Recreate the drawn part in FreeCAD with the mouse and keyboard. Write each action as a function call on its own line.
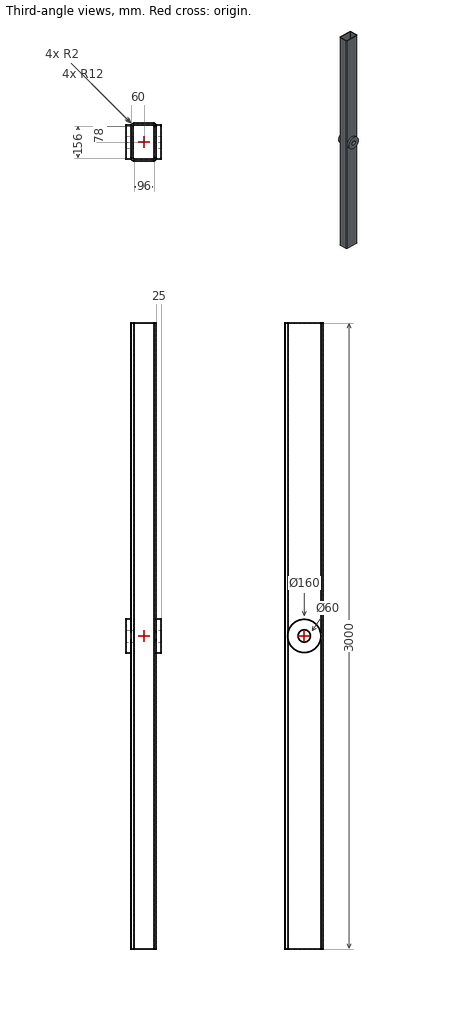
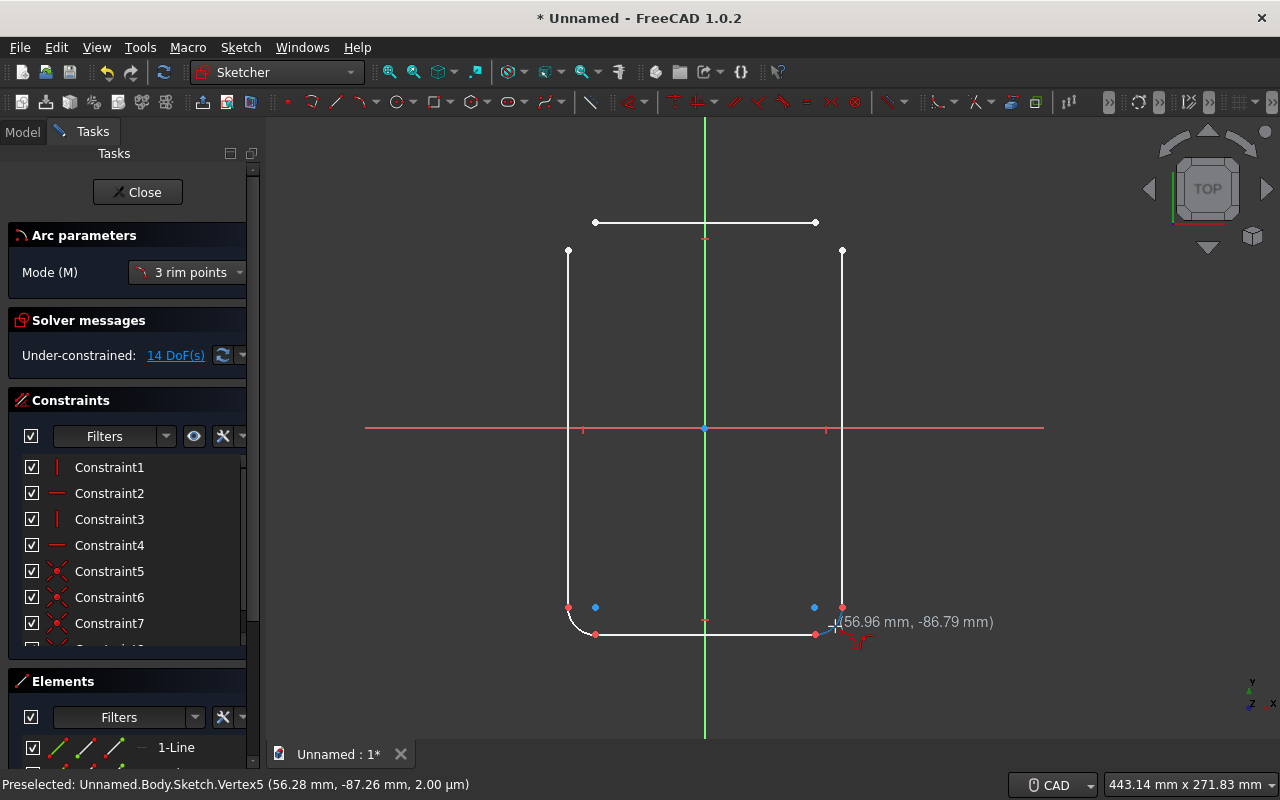
click(842, 251)
click(815, 223)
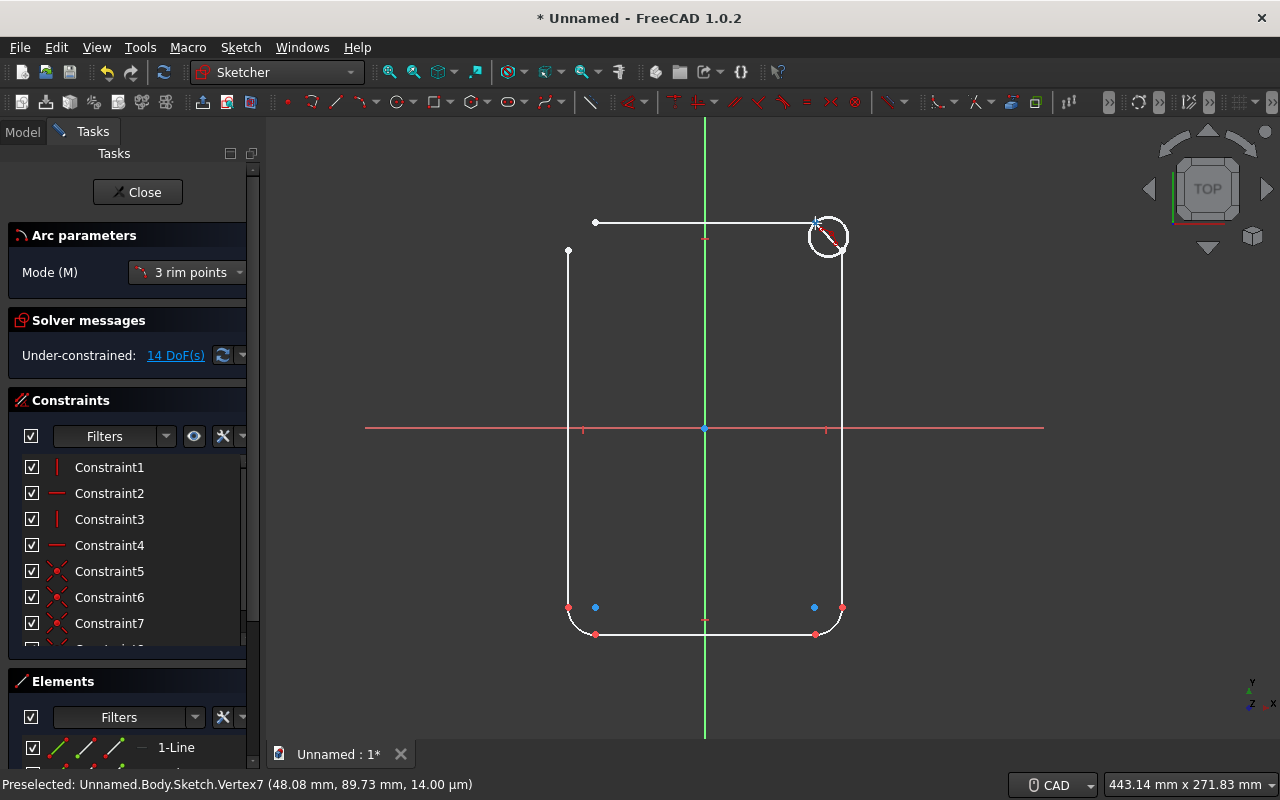
scroll(834, 230, up, 4)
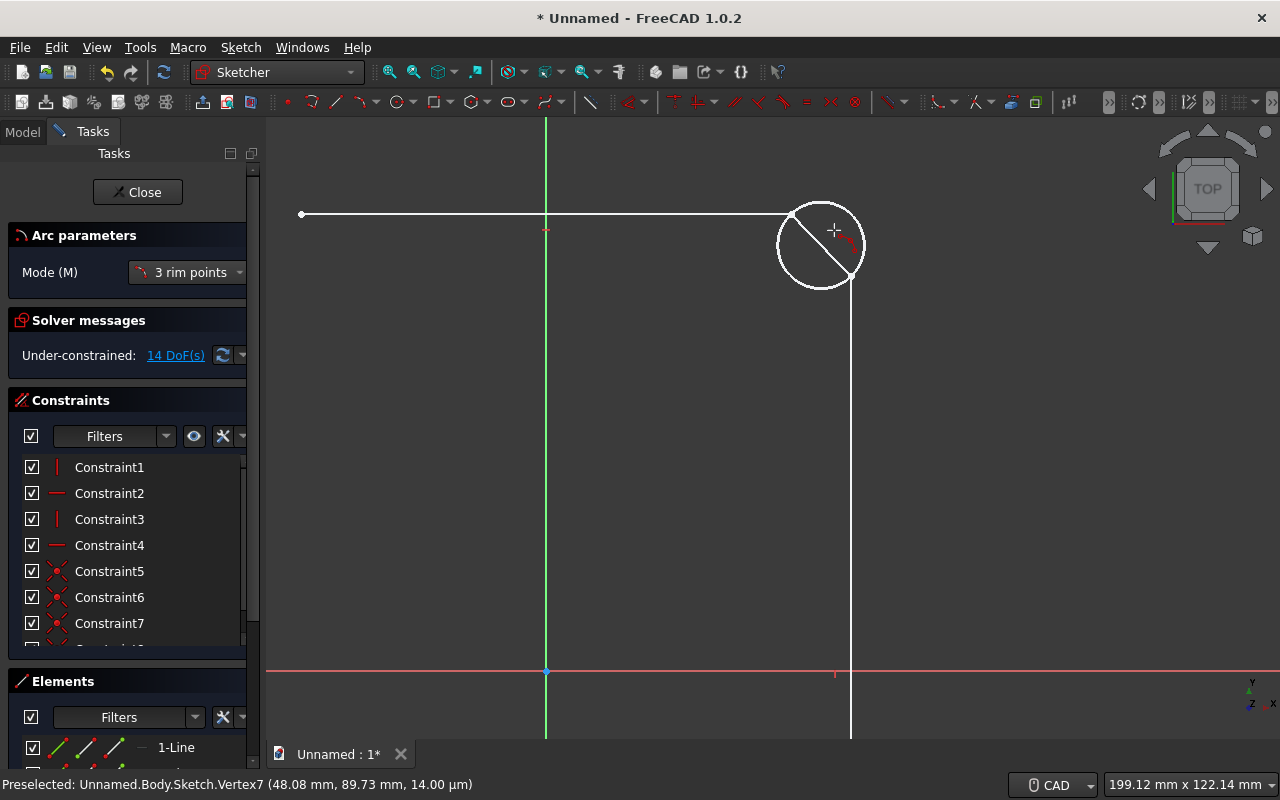
click(834, 231)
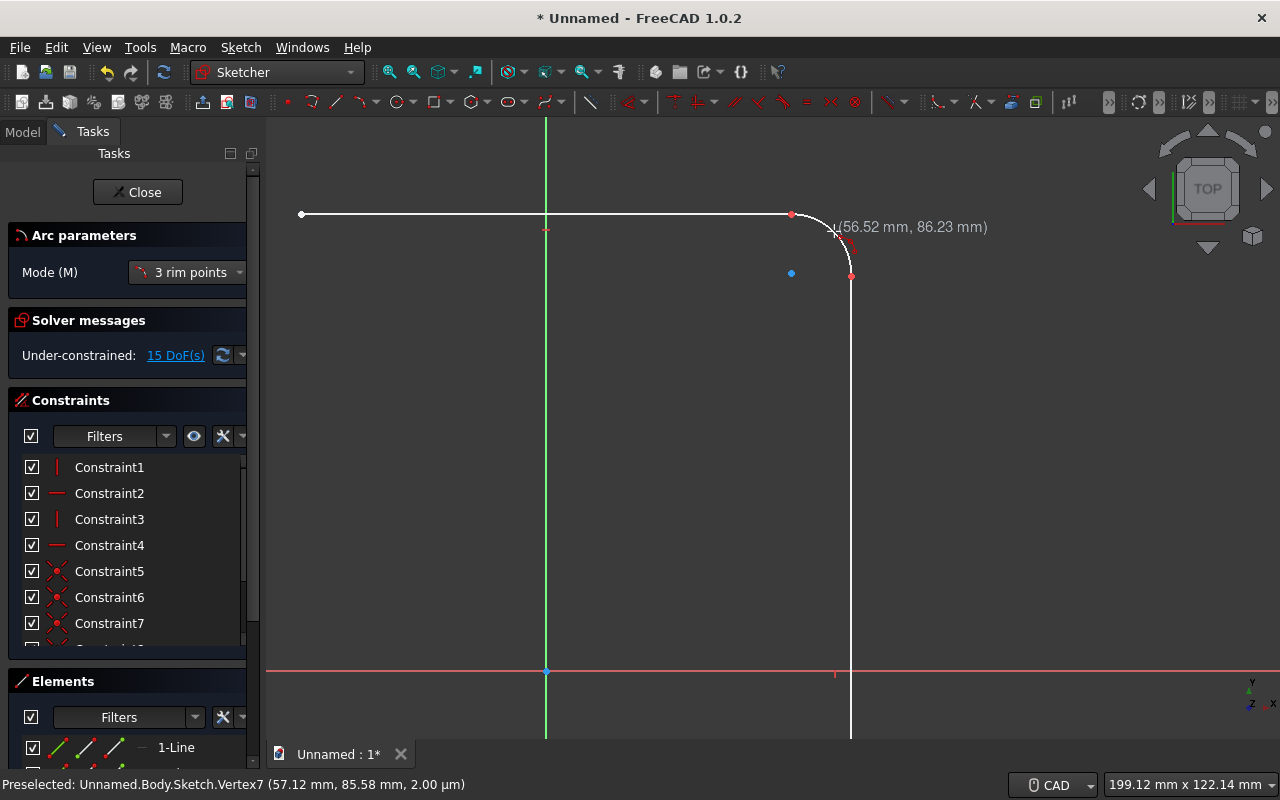
click(301, 214)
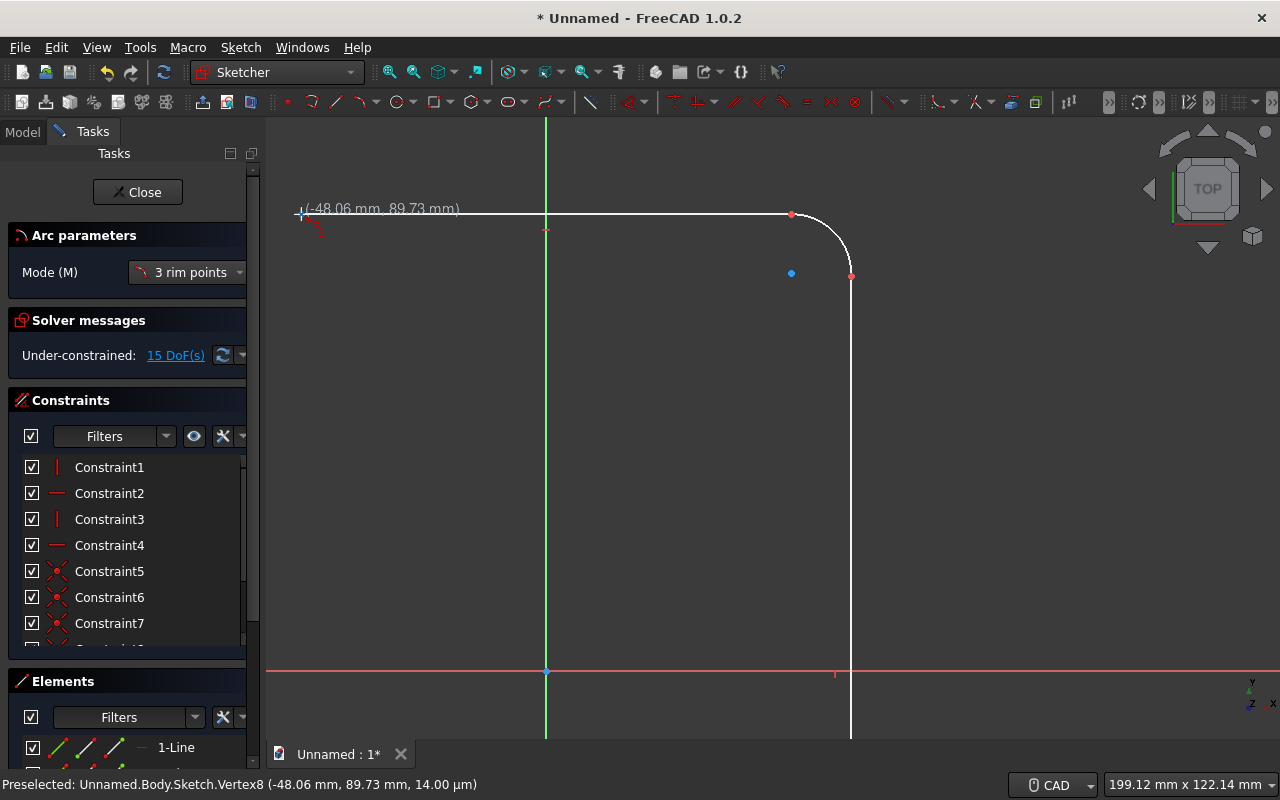
scroll(834, 230, down, 4)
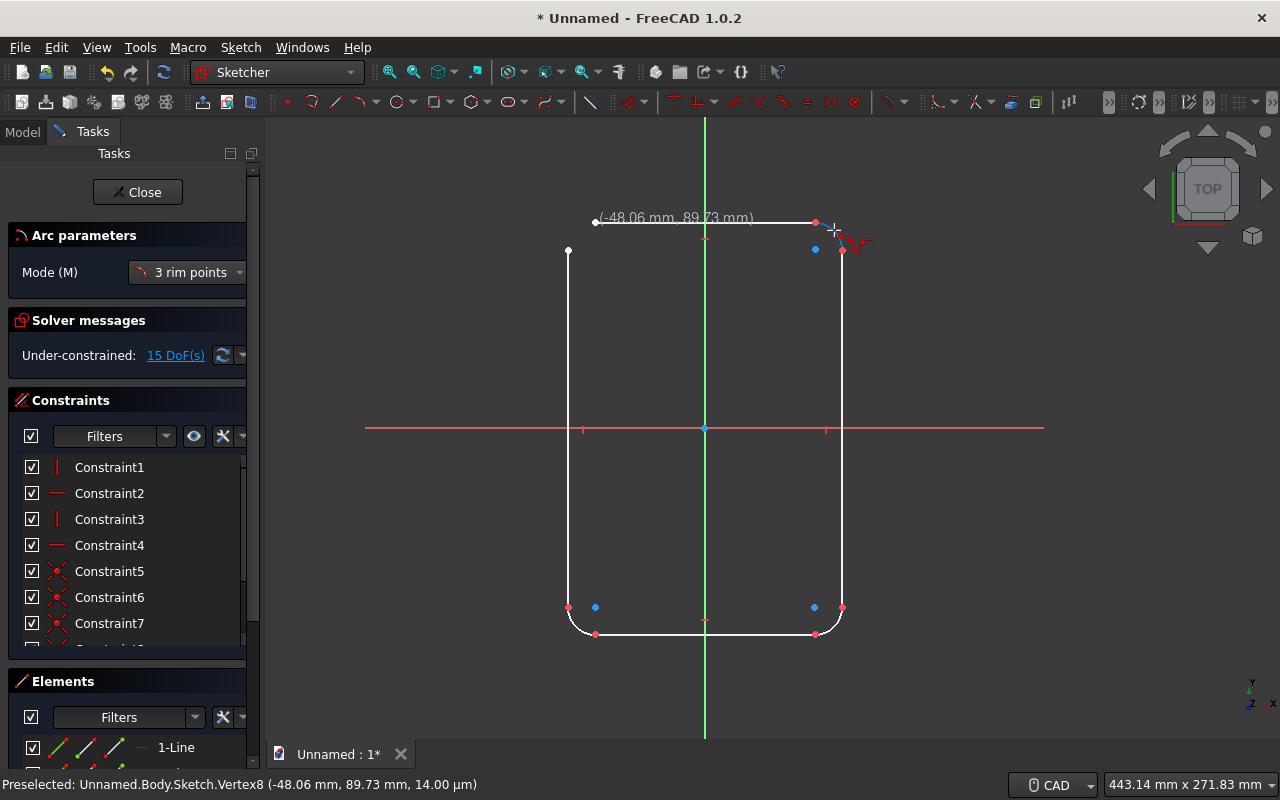
click(568, 251)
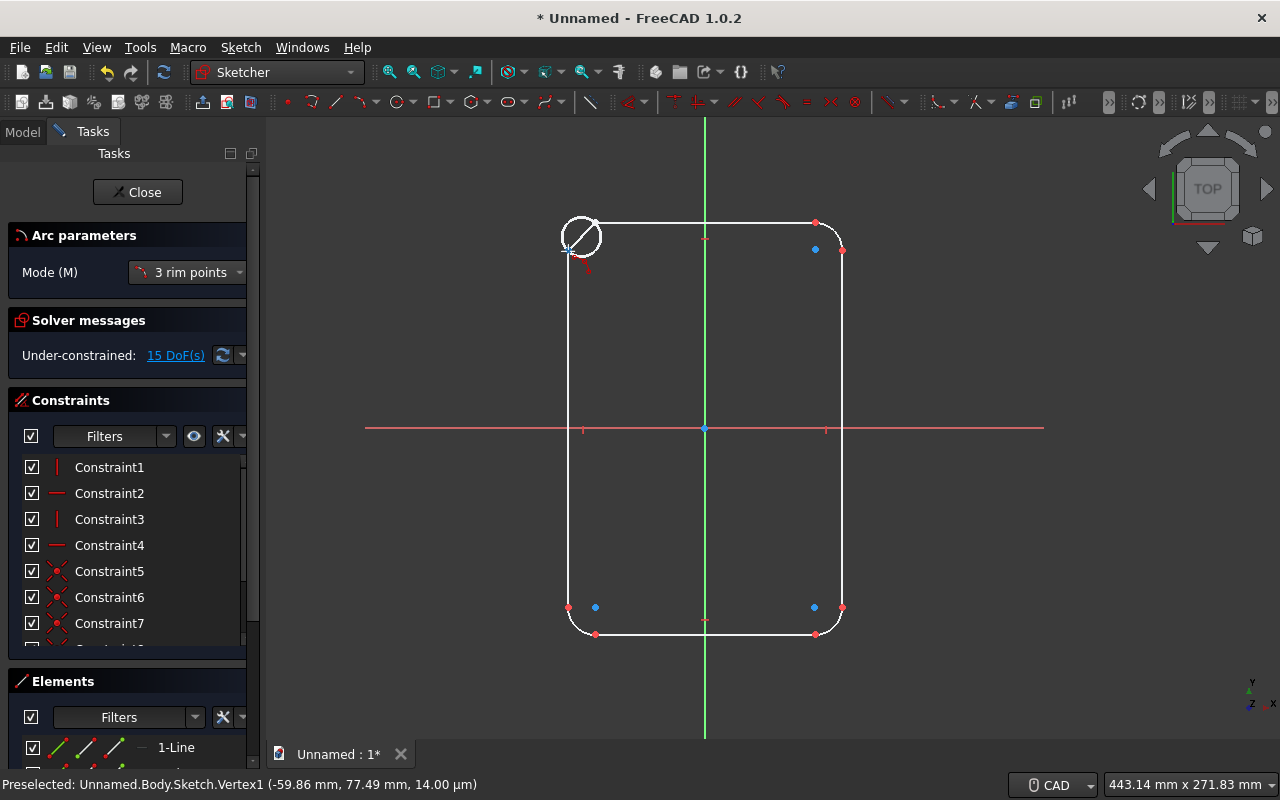
scroll(576, 230, up, 4)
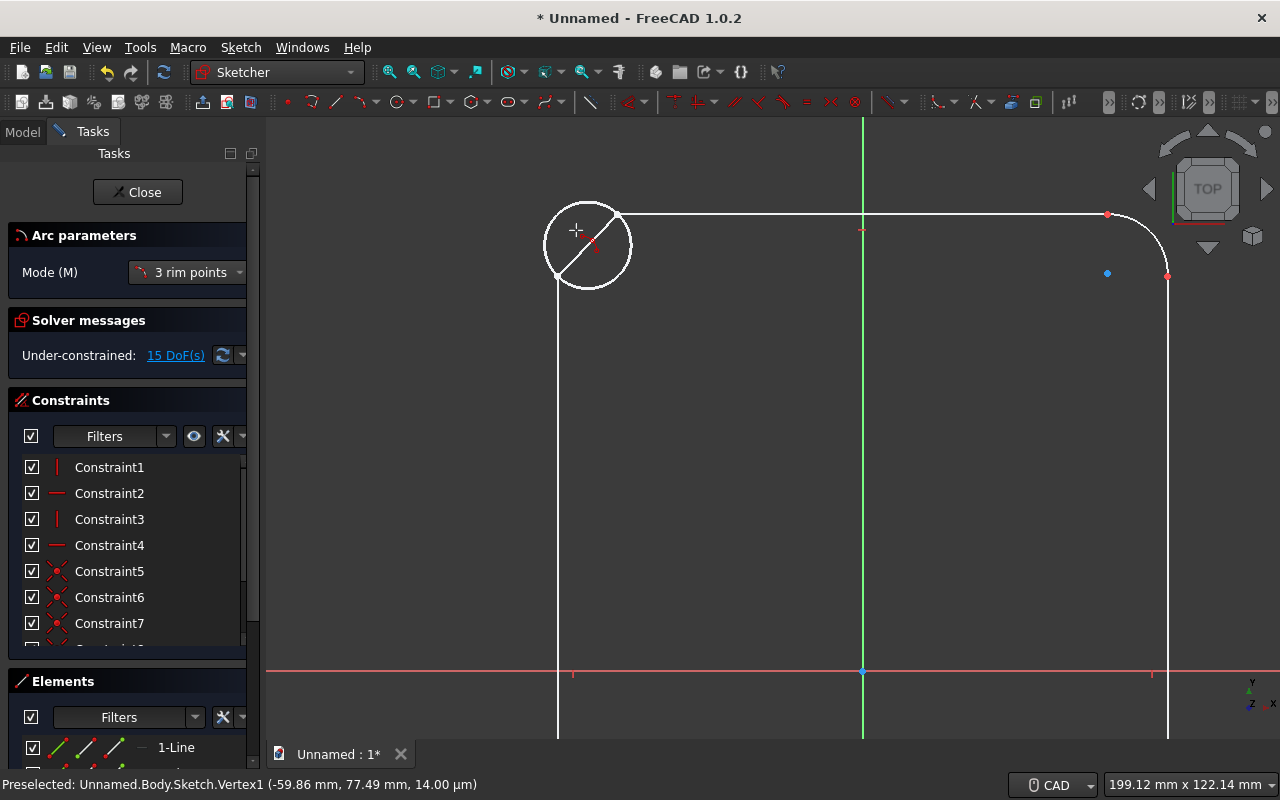
click(575, 231)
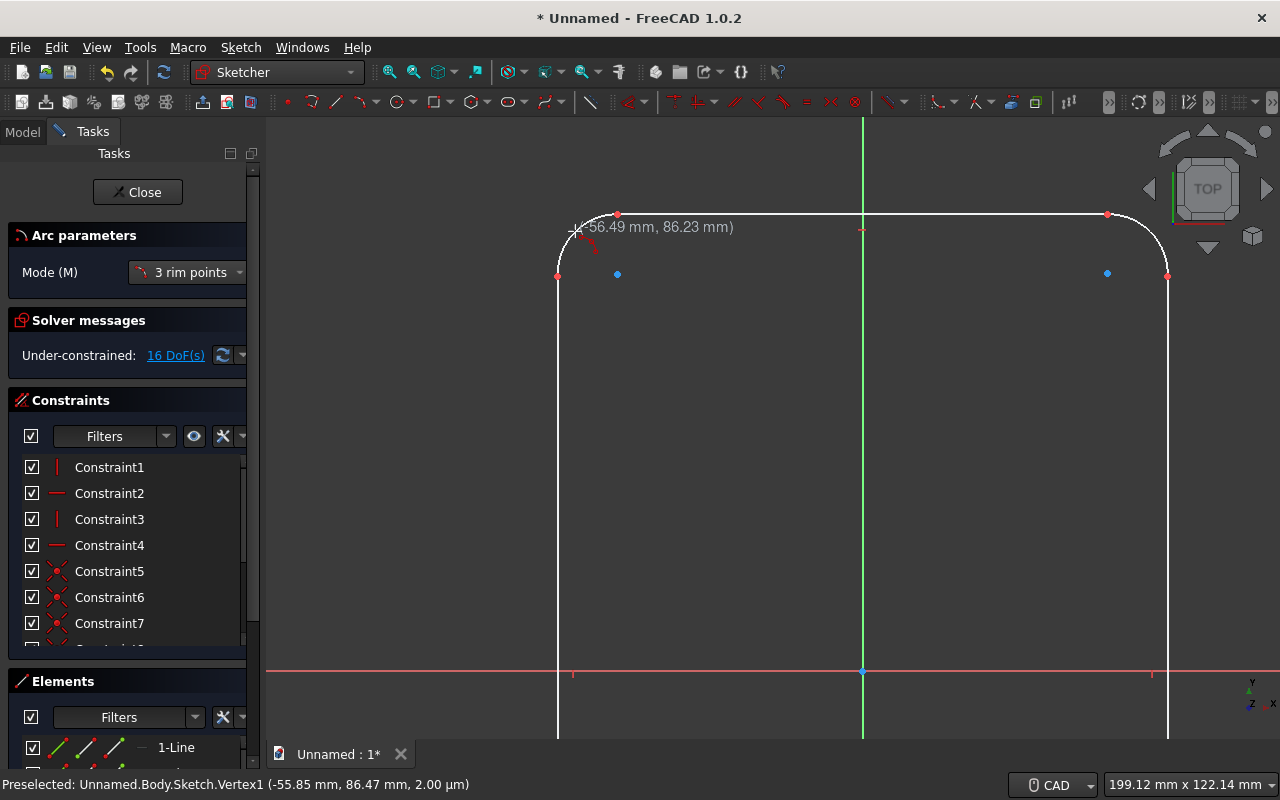
click(336, 102)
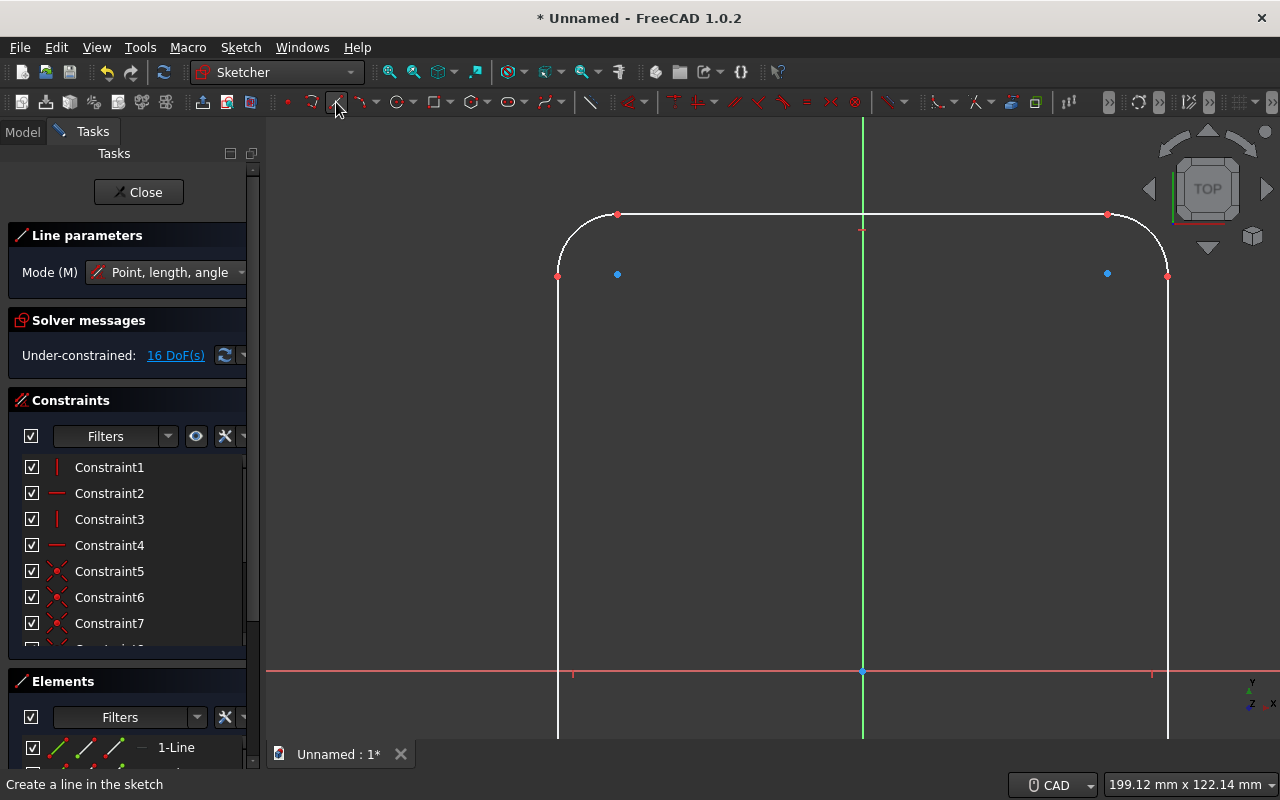
scroll(618, 264, up, 3)